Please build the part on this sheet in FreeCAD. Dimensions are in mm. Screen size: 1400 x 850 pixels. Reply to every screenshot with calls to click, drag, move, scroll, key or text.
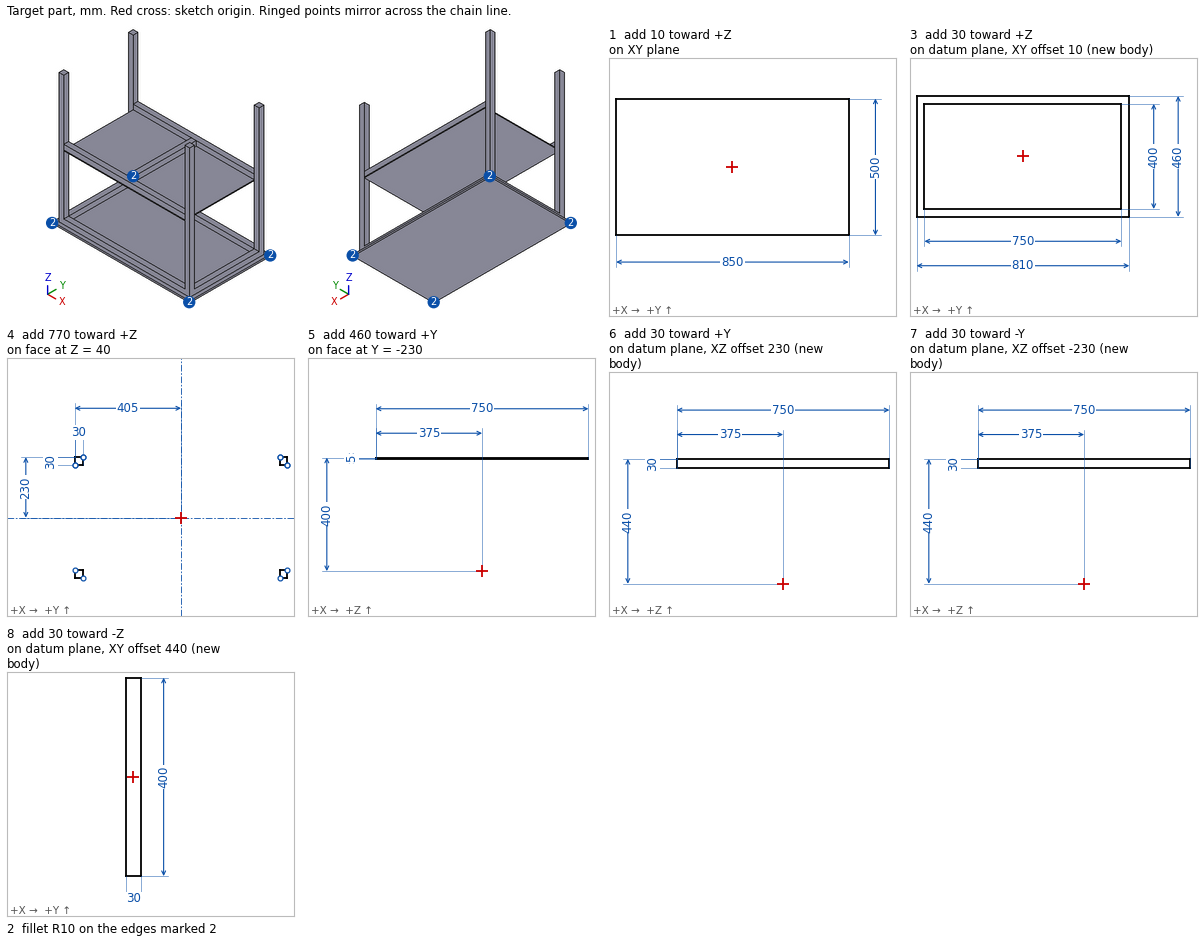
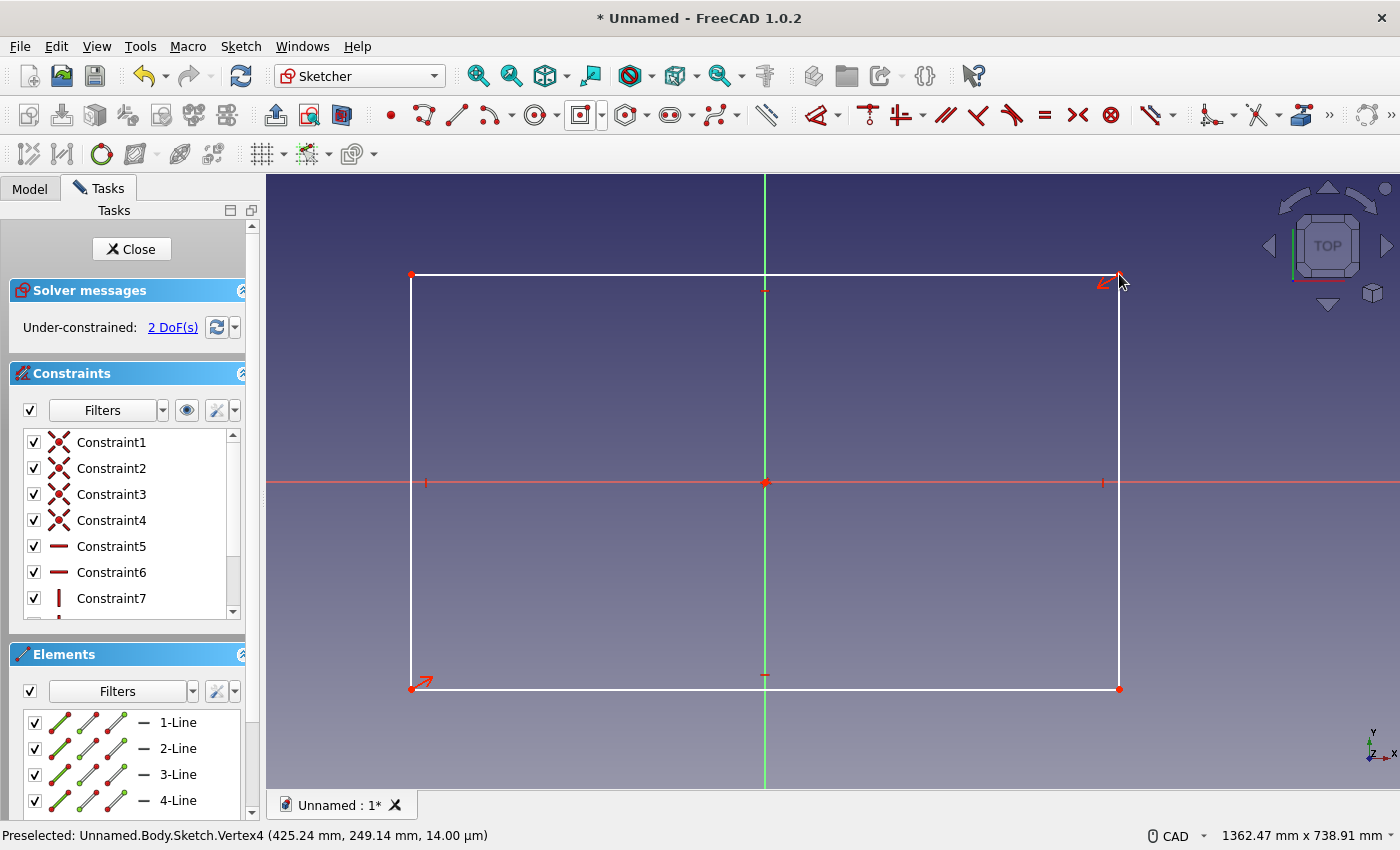
click(623, 690)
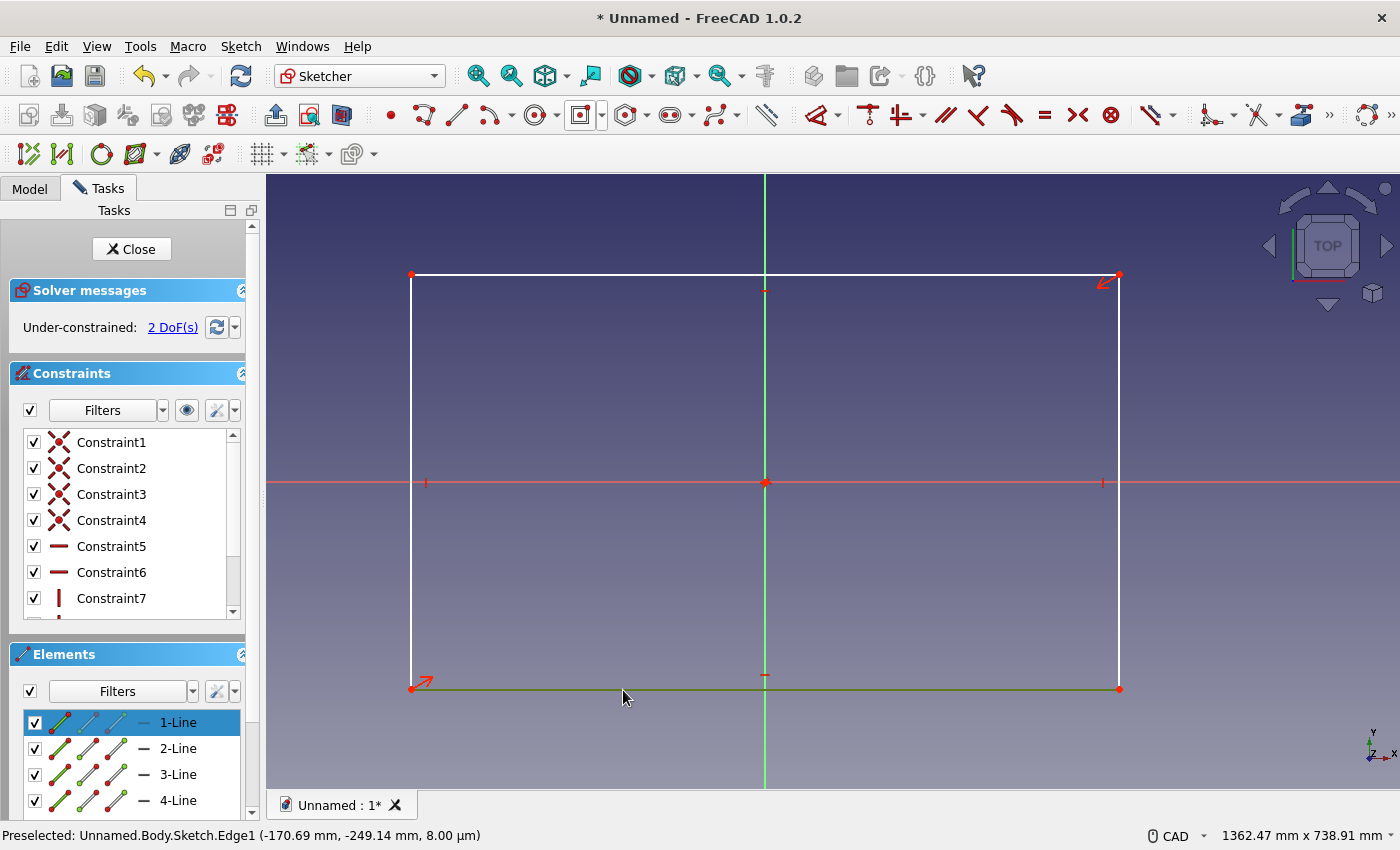
click(838, 116)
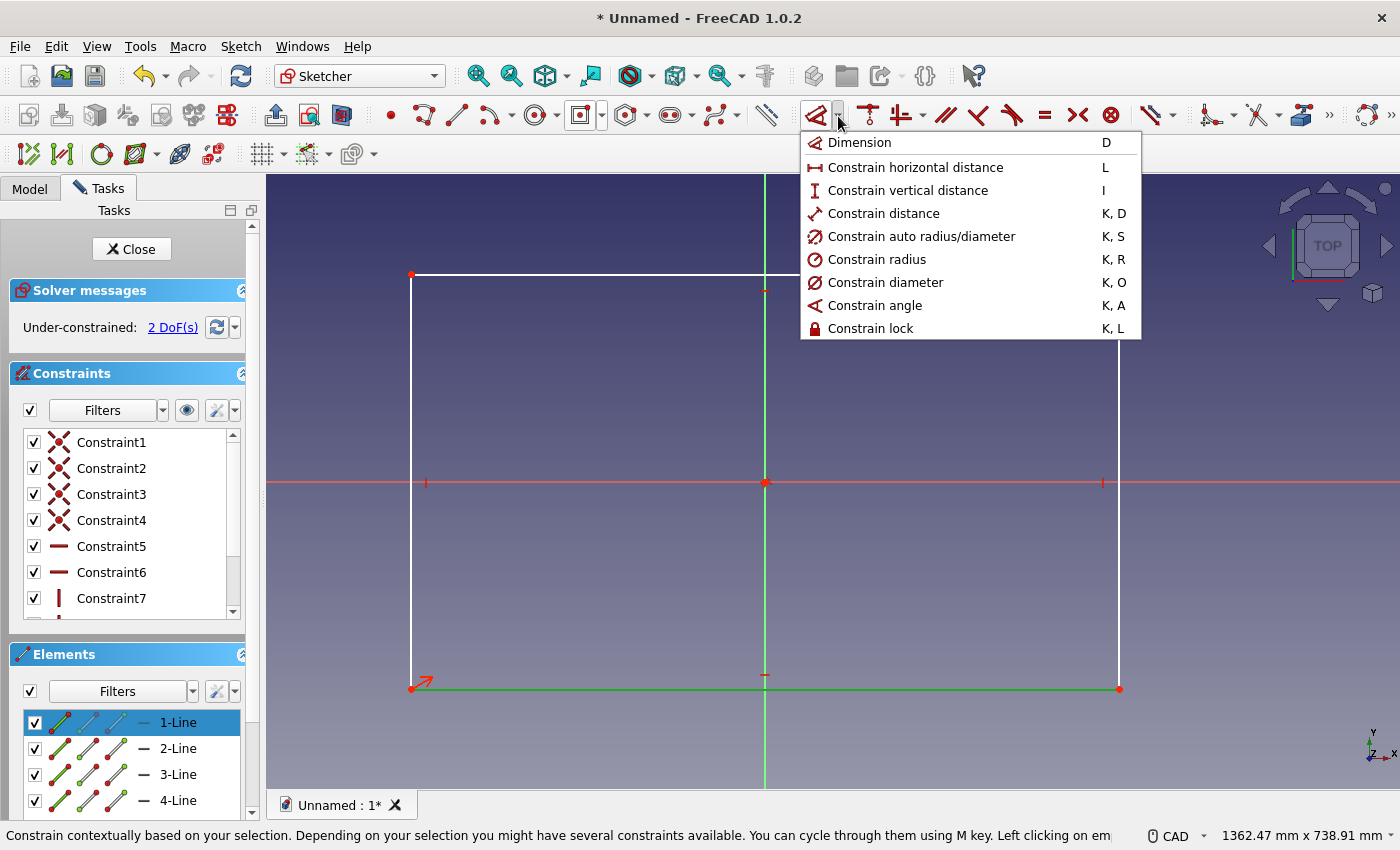
click(971, 168)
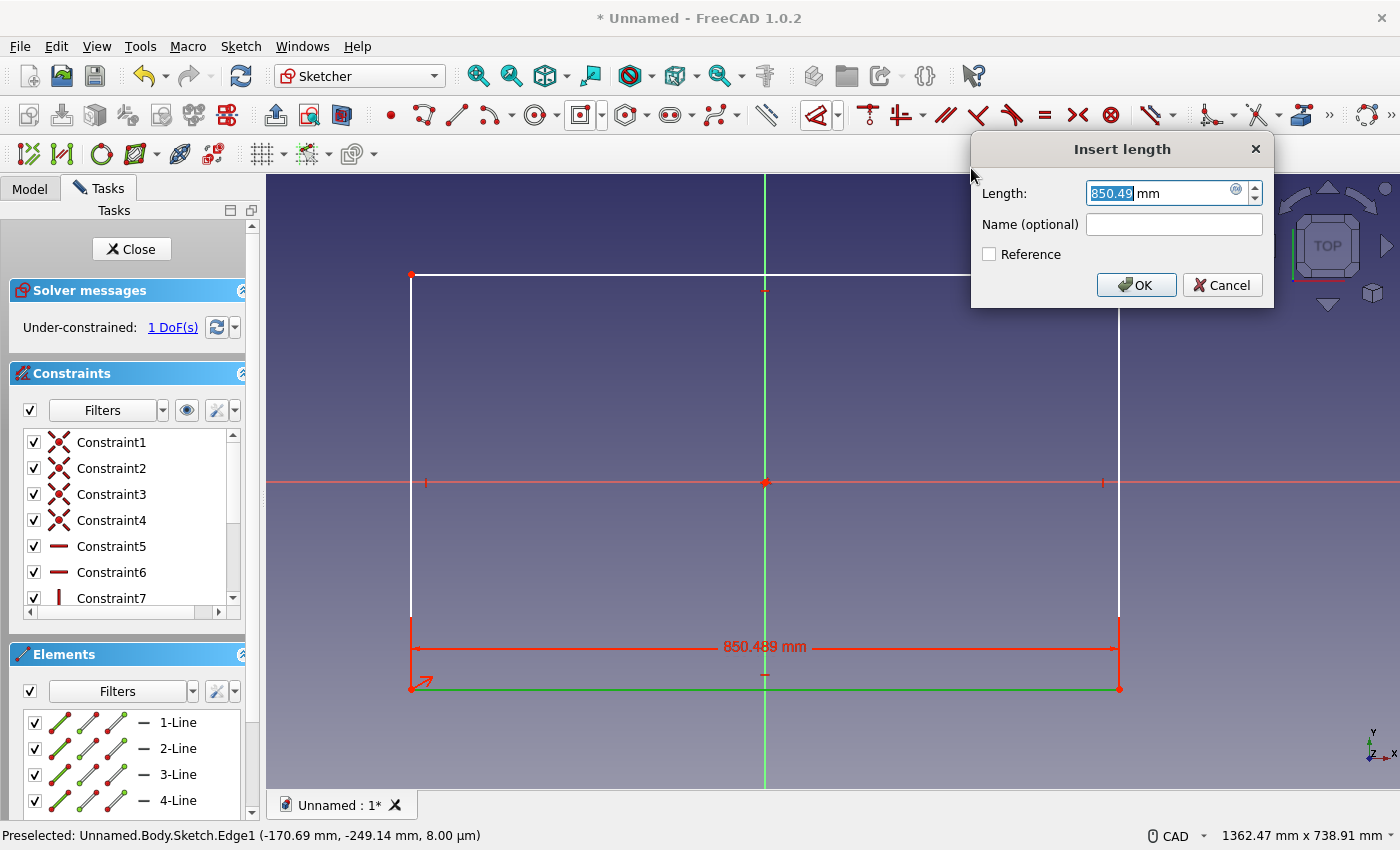
text(850)
key(Return)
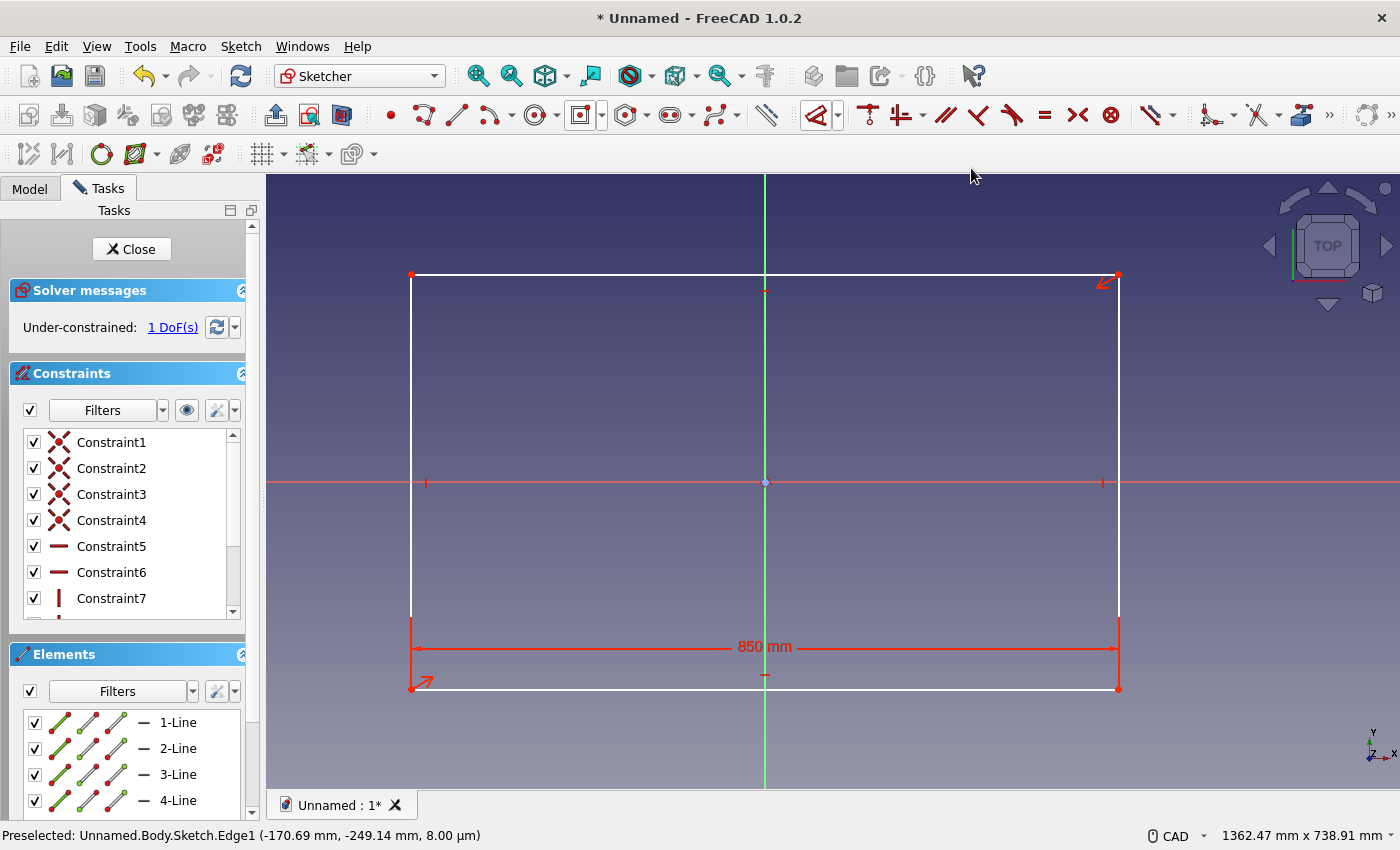
click(1119, 565)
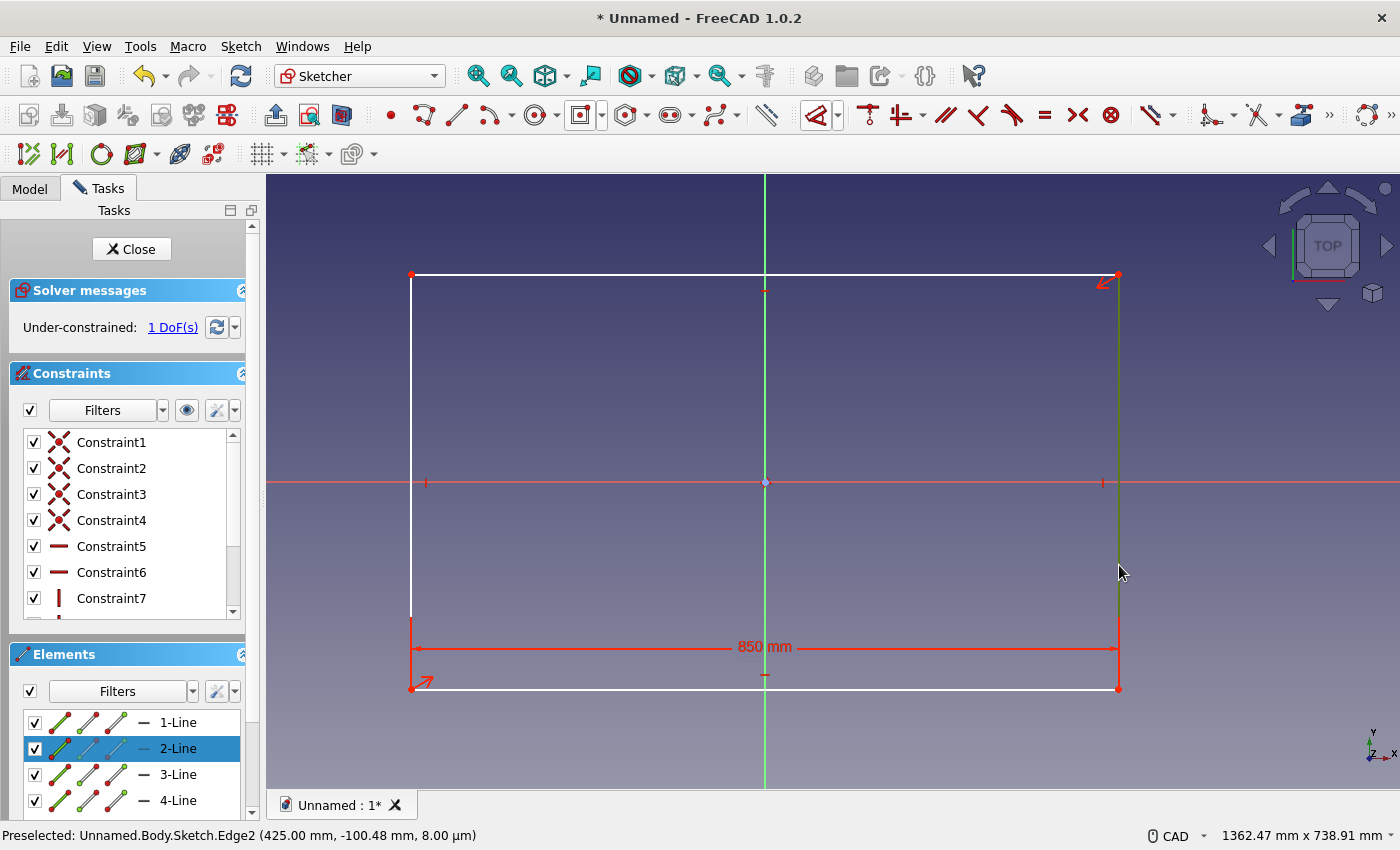
key(i)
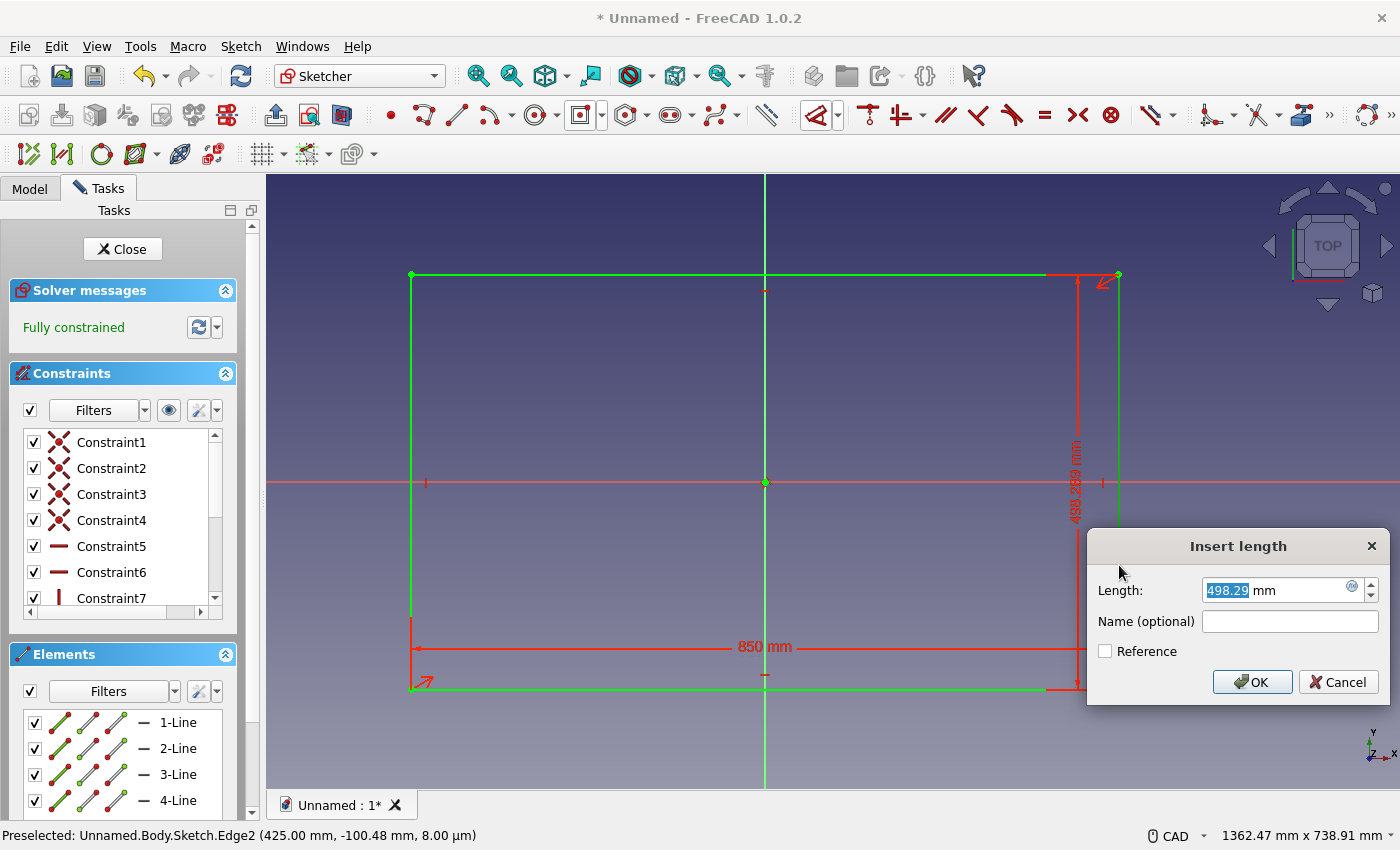
text(500)
key(Return)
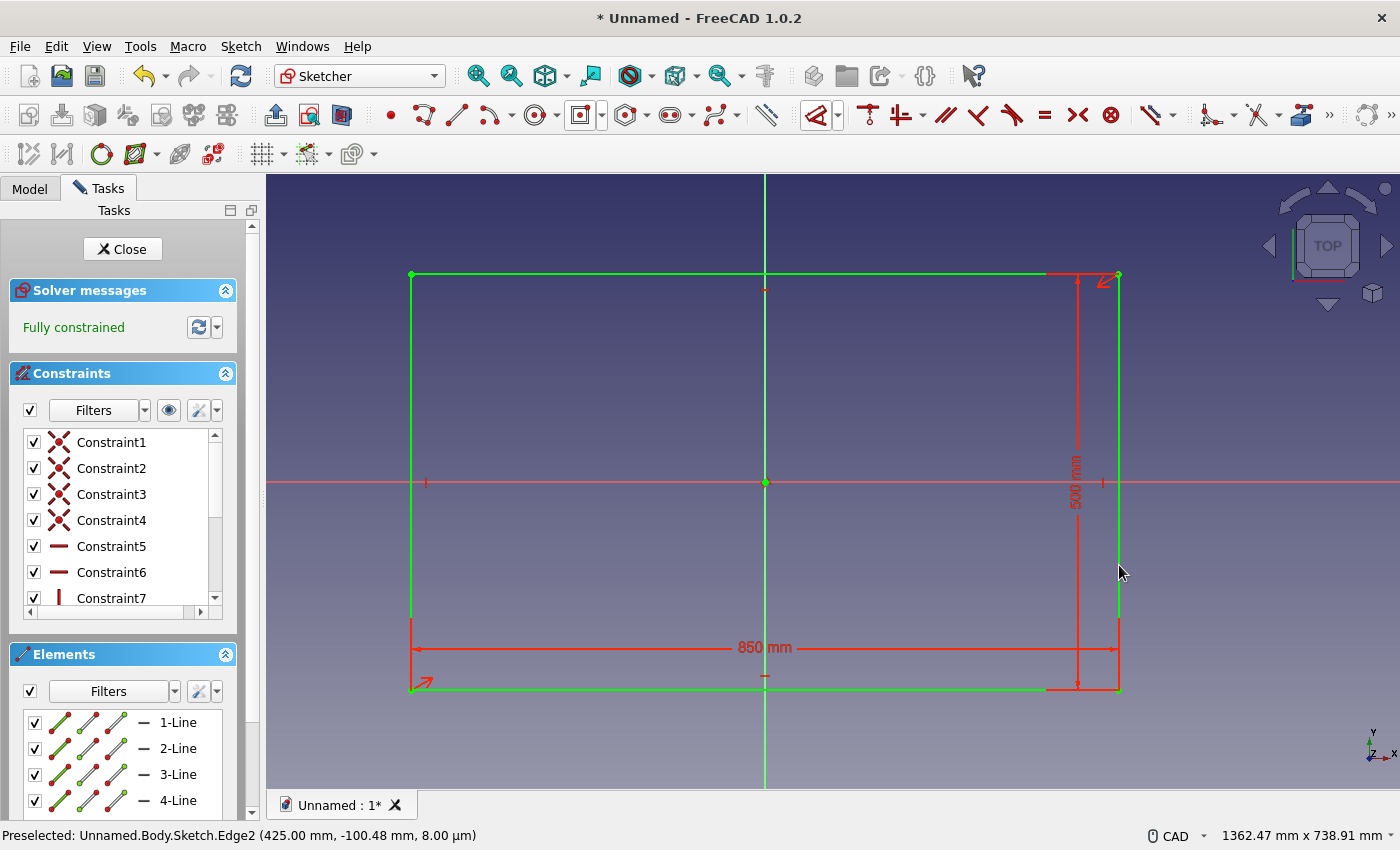
click(123, 249)